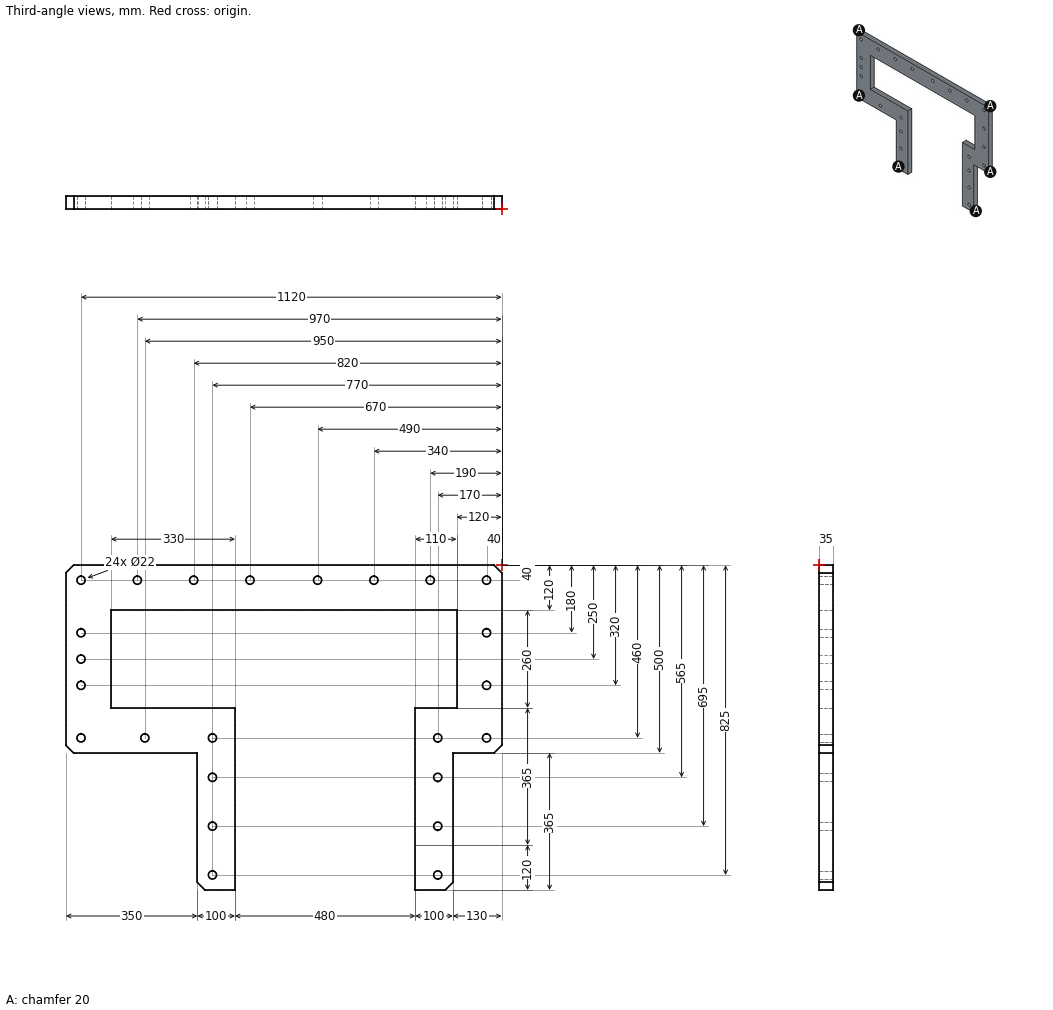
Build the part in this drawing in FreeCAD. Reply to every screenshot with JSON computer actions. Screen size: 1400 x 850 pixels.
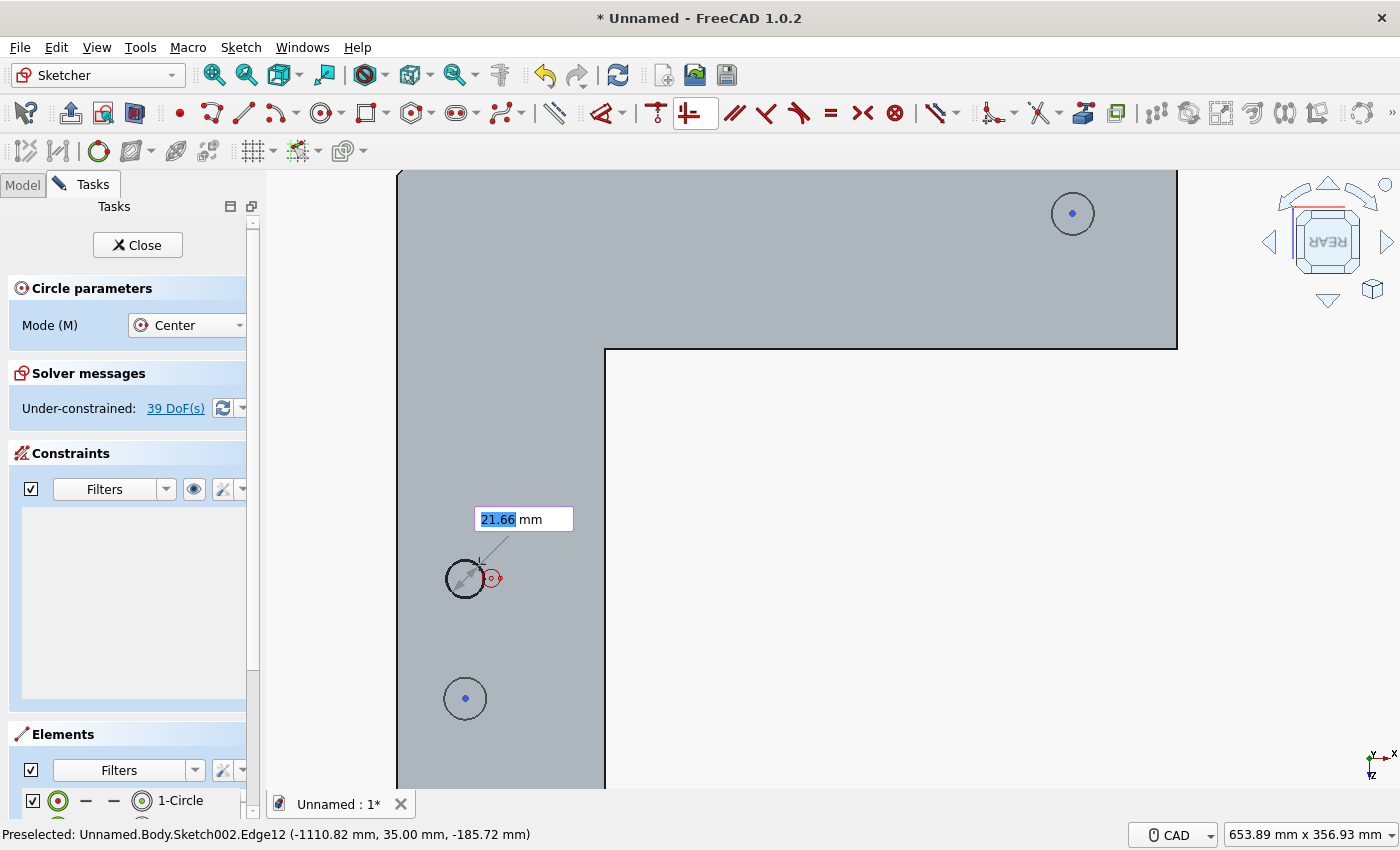
{"action": "left_click", "coordinate": [480, 561]}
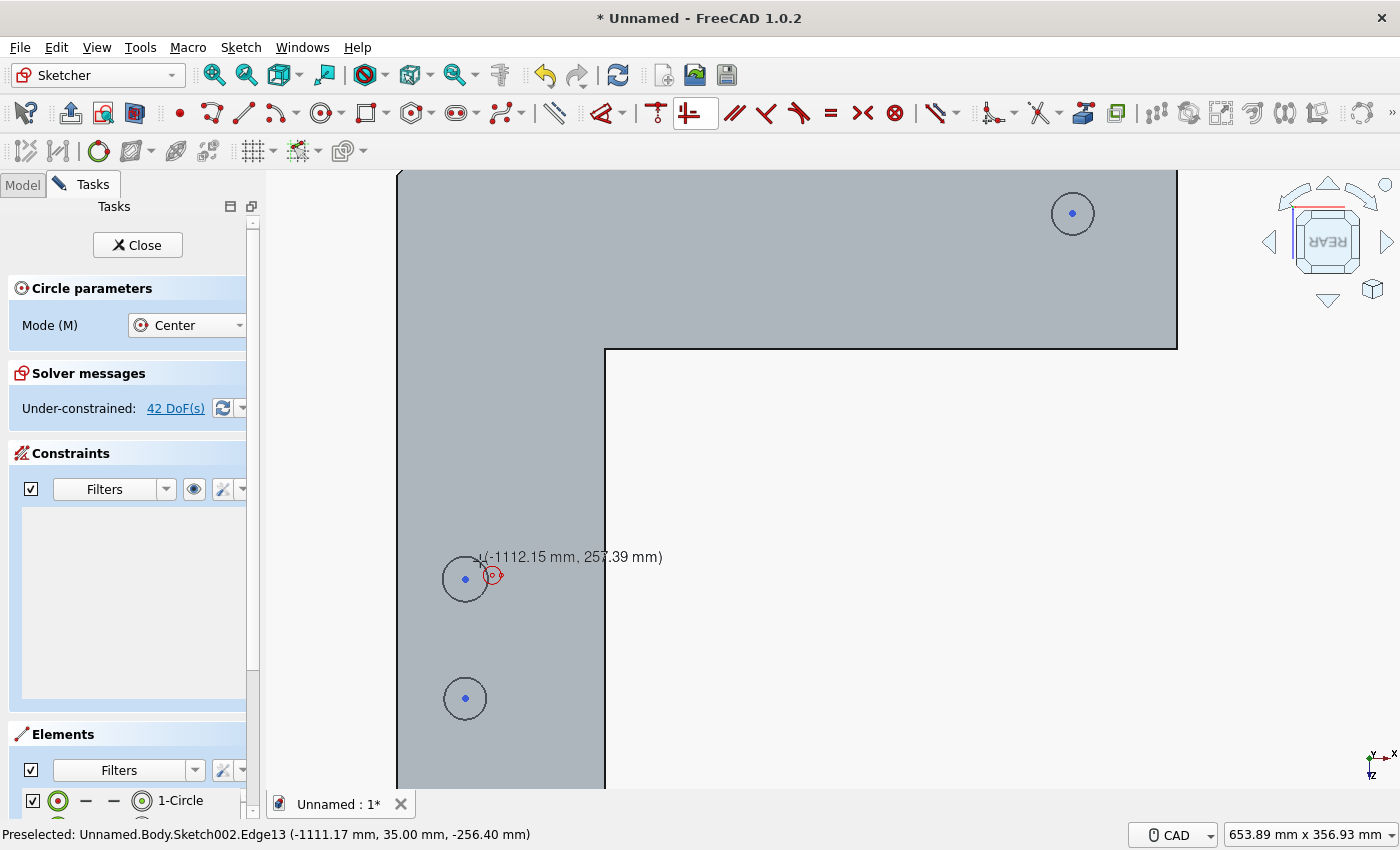
{"action": "scroll", "coordinate": [479, 564], "scroll_direction": "down", "scroll_amount": 6}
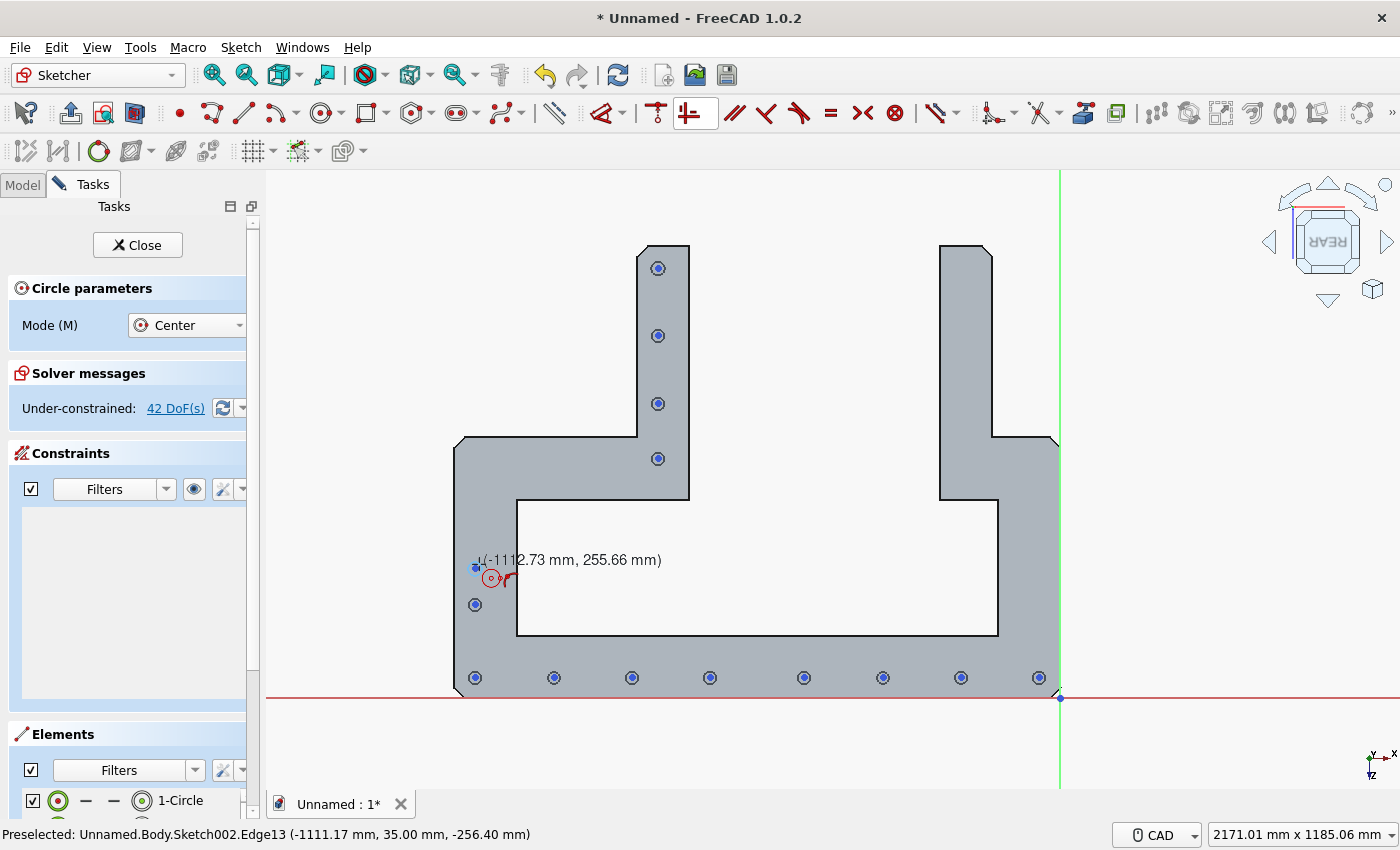
{"action": "left_click", "coordinate": [475, 531]}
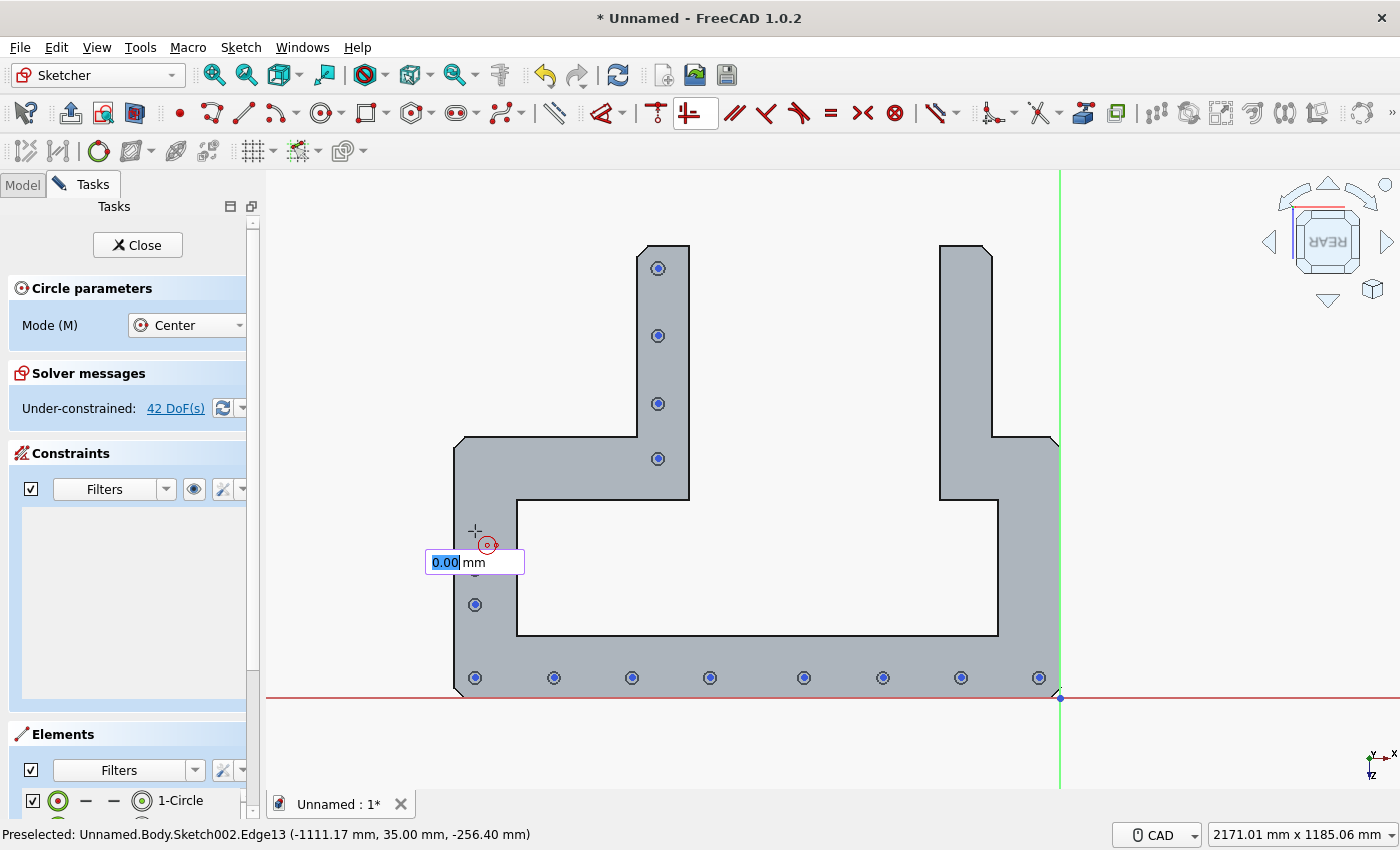
{"action": "scroll", "coordinate": [479, 527], "scroll_direction": "up", "scroll_amount": 6}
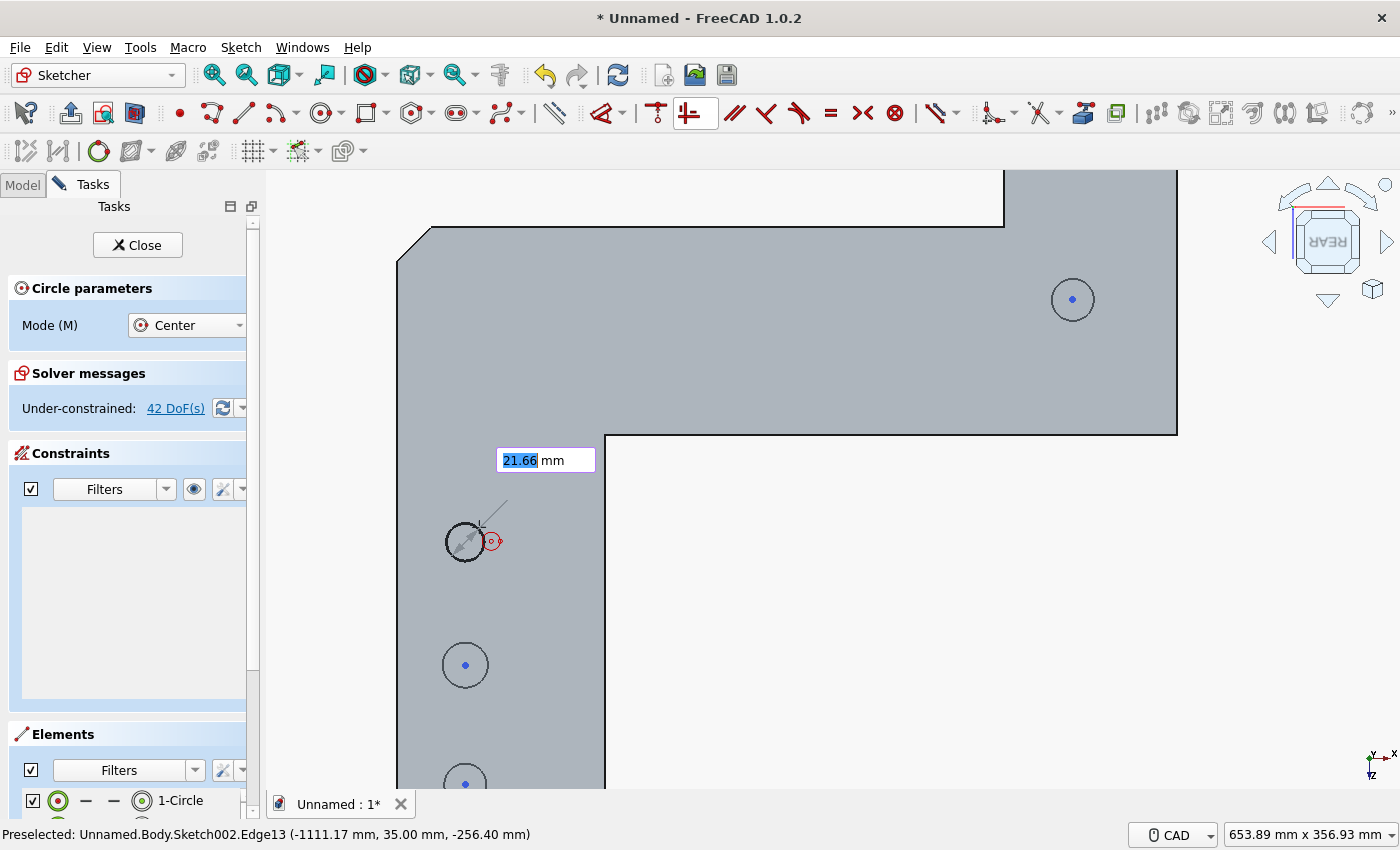
{"action": "left_click", "coordinate": [480, 526]}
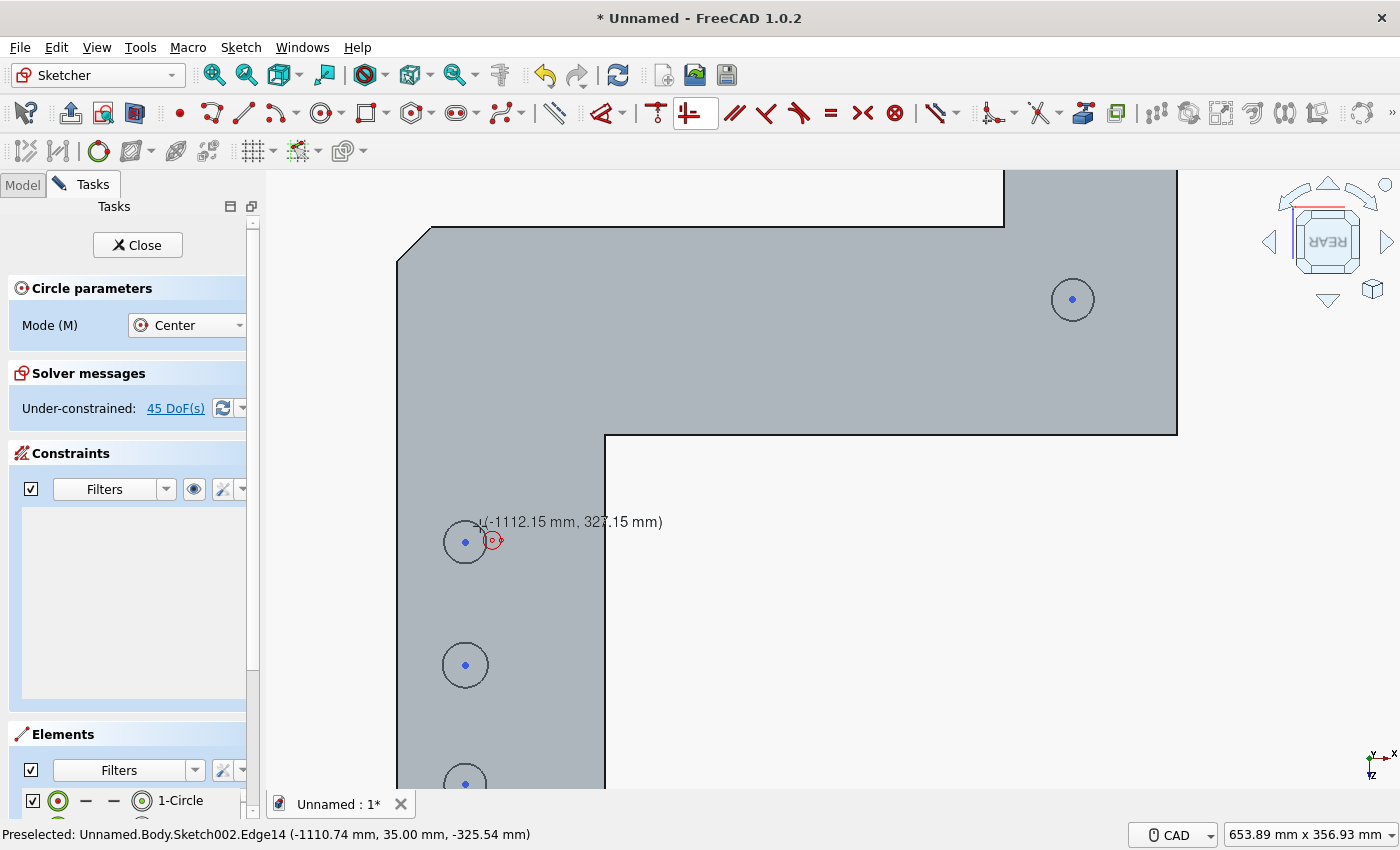
{"action": "scroll", "coordinate": [479, 527], "scroll_direction": "down", "scroll_amount": 6}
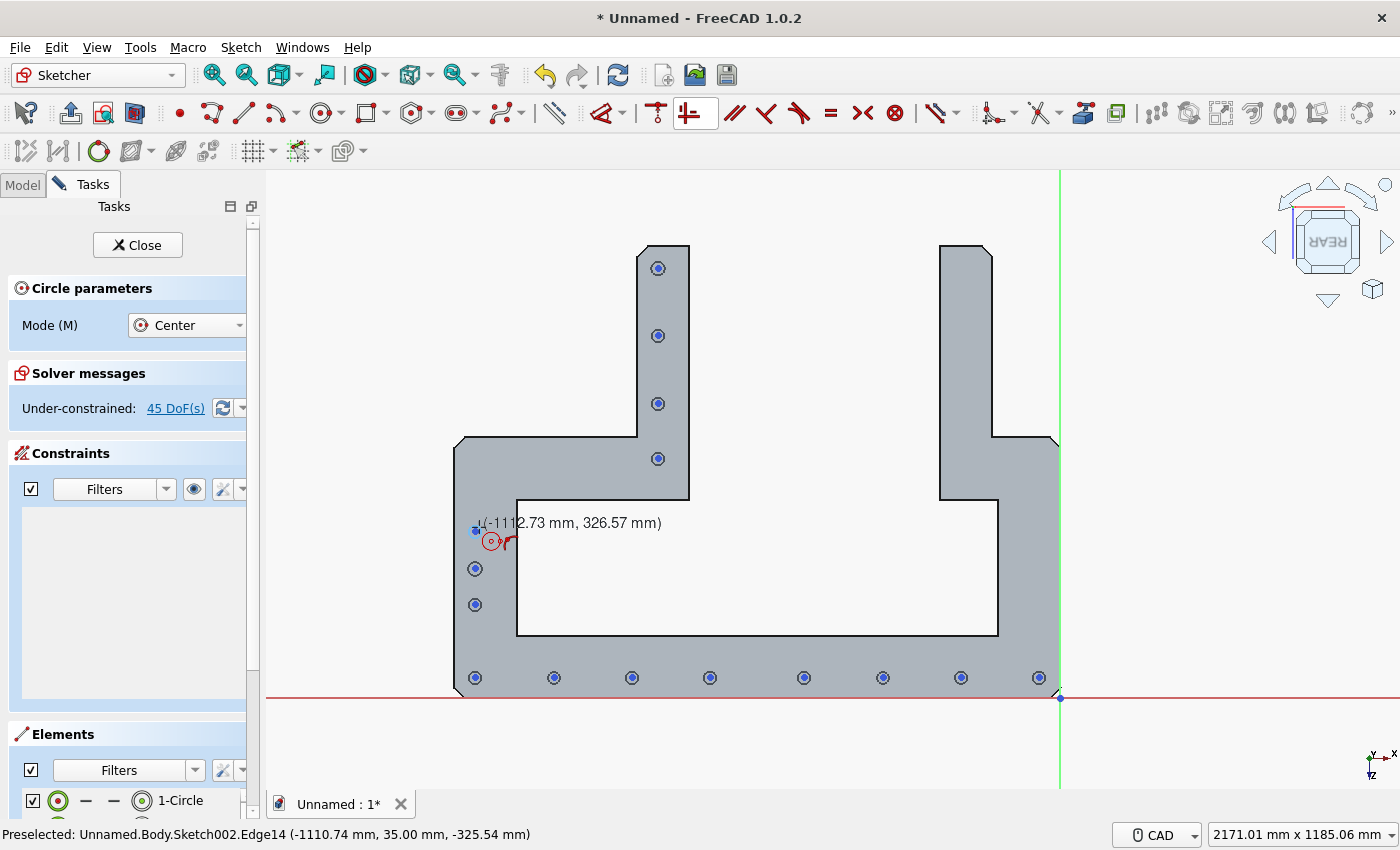
{"action": "left_click", "coordinate": [475, 458]}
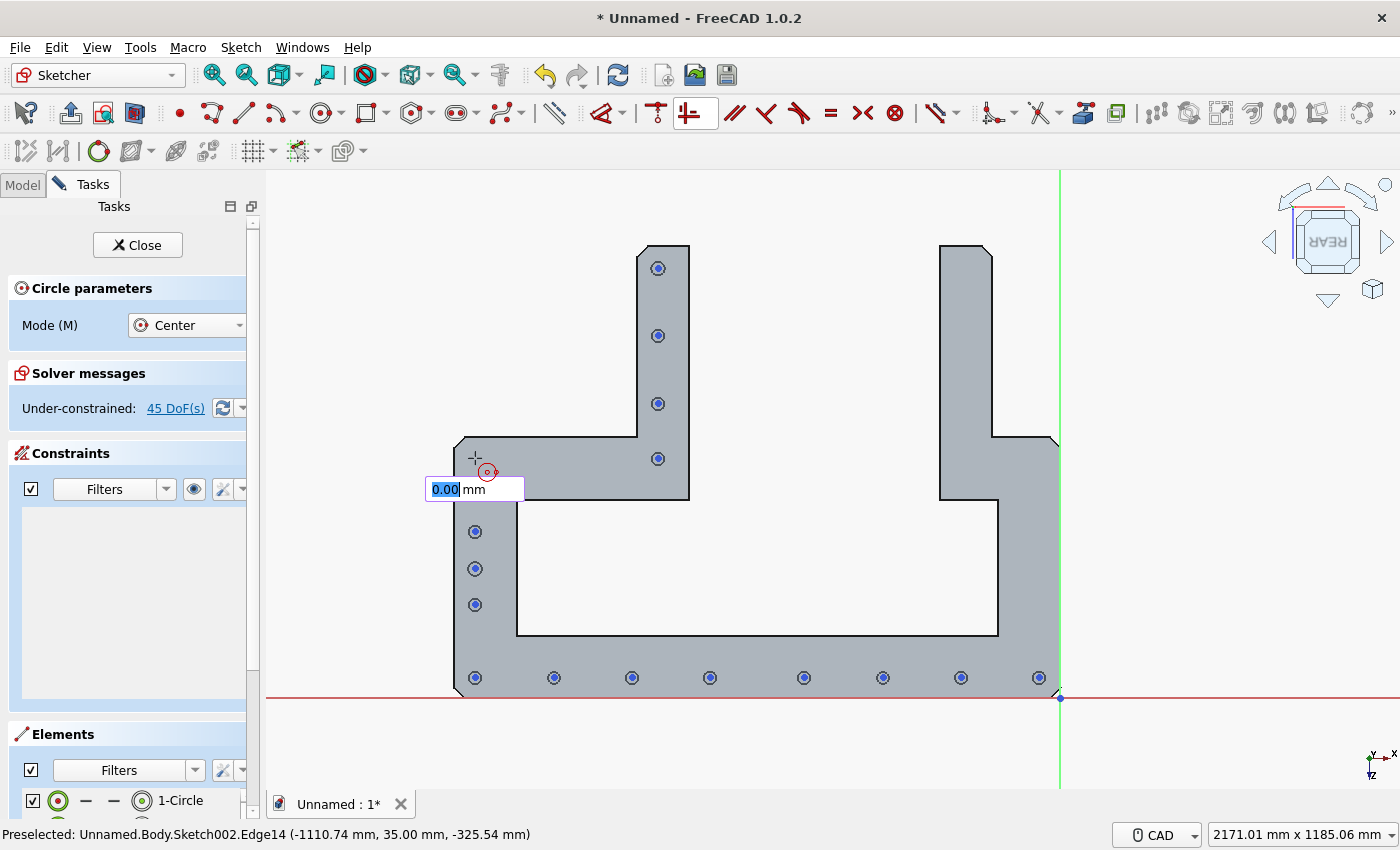
{"action": "scroll", "coordinate": [479, 454], "scroll_direction": "up", "scroll_amount": 6}